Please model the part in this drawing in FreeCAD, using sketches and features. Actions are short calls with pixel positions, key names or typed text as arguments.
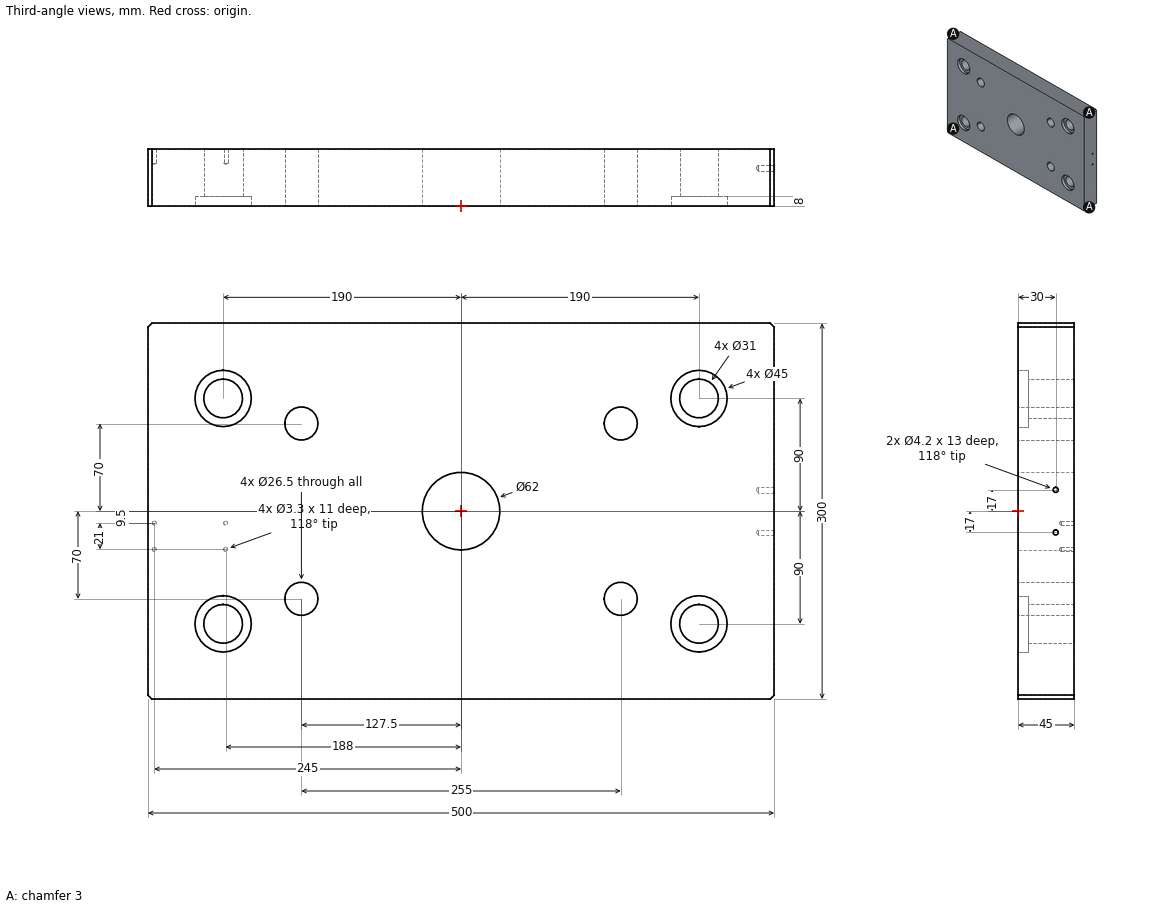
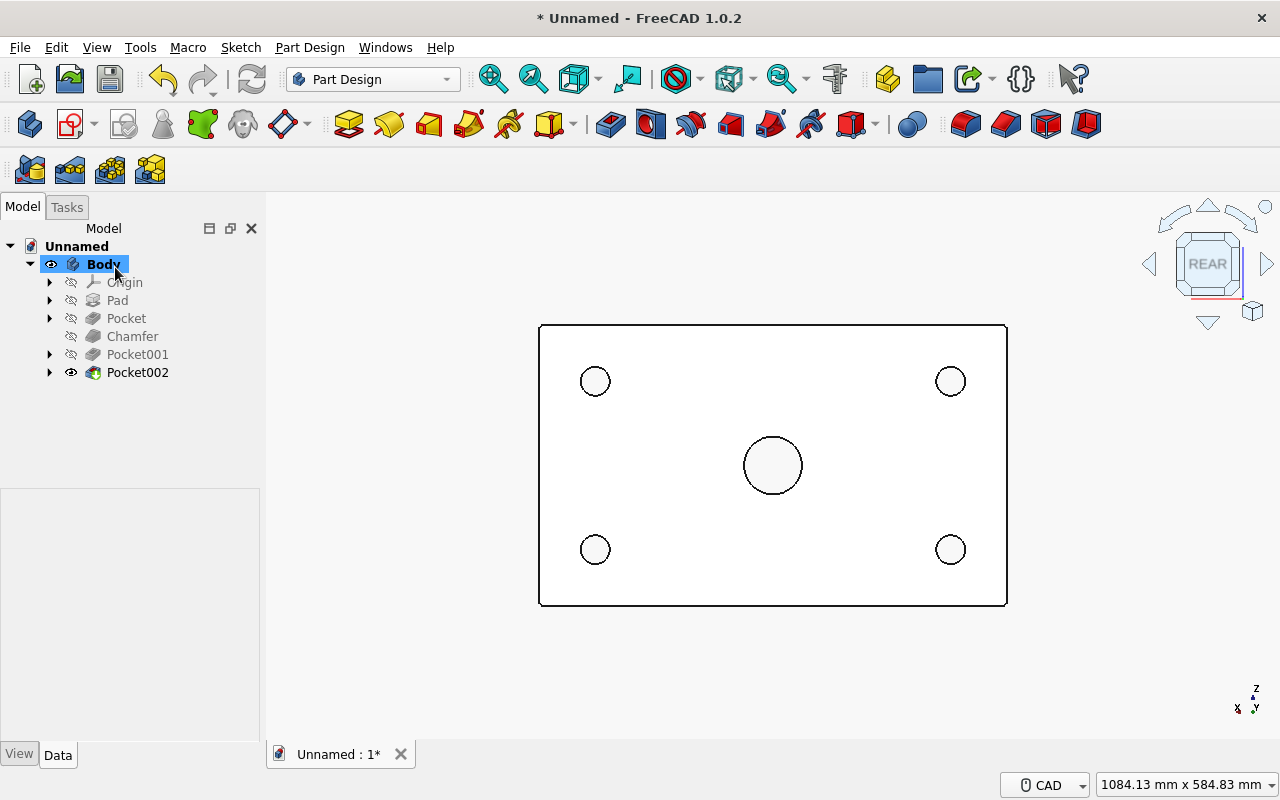
click(907, 465)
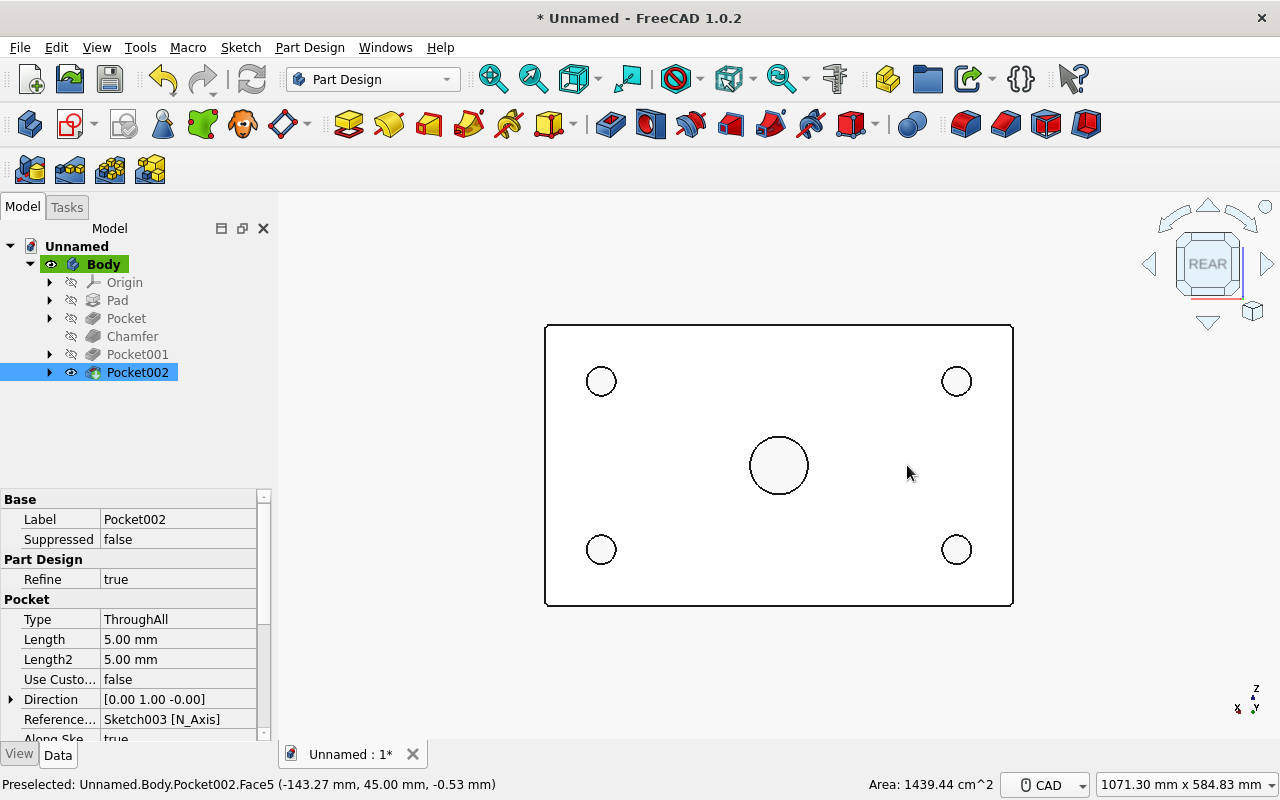
click(70, 124)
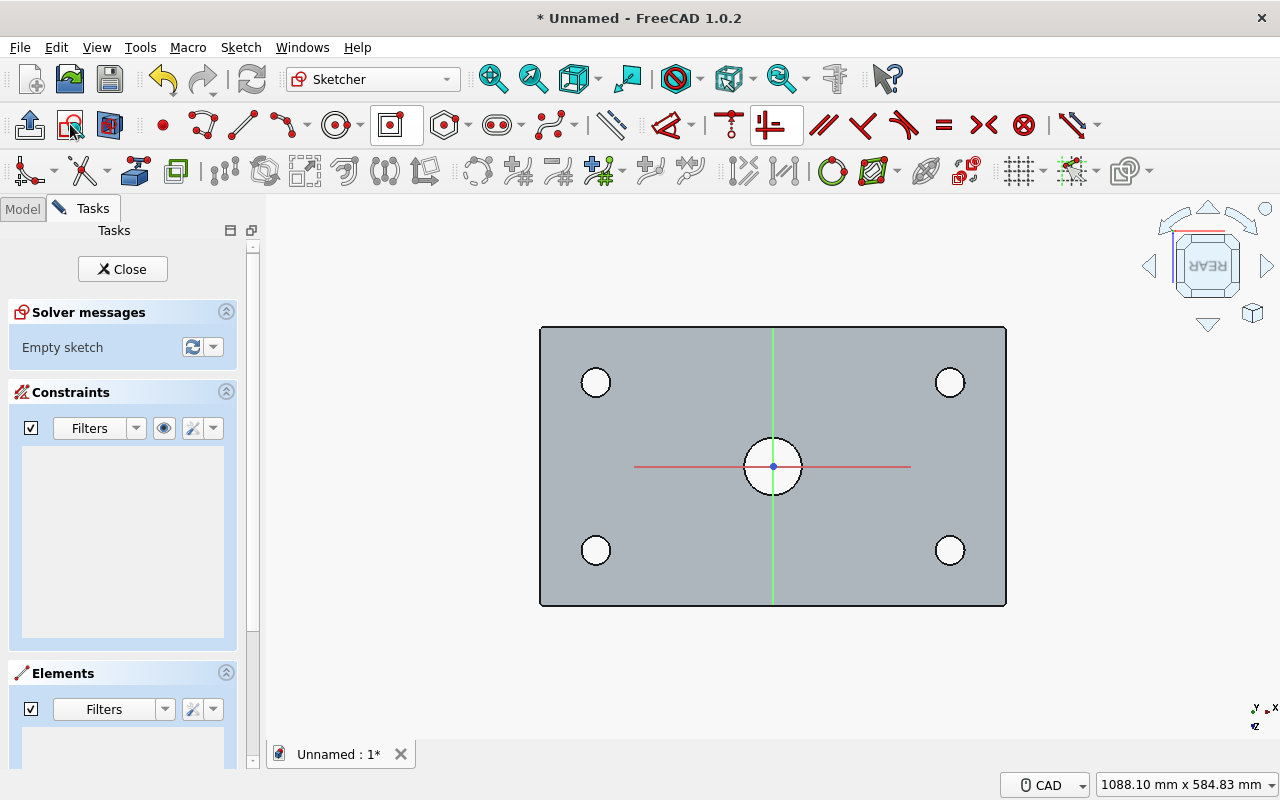
scroll(558, 446, up, 12)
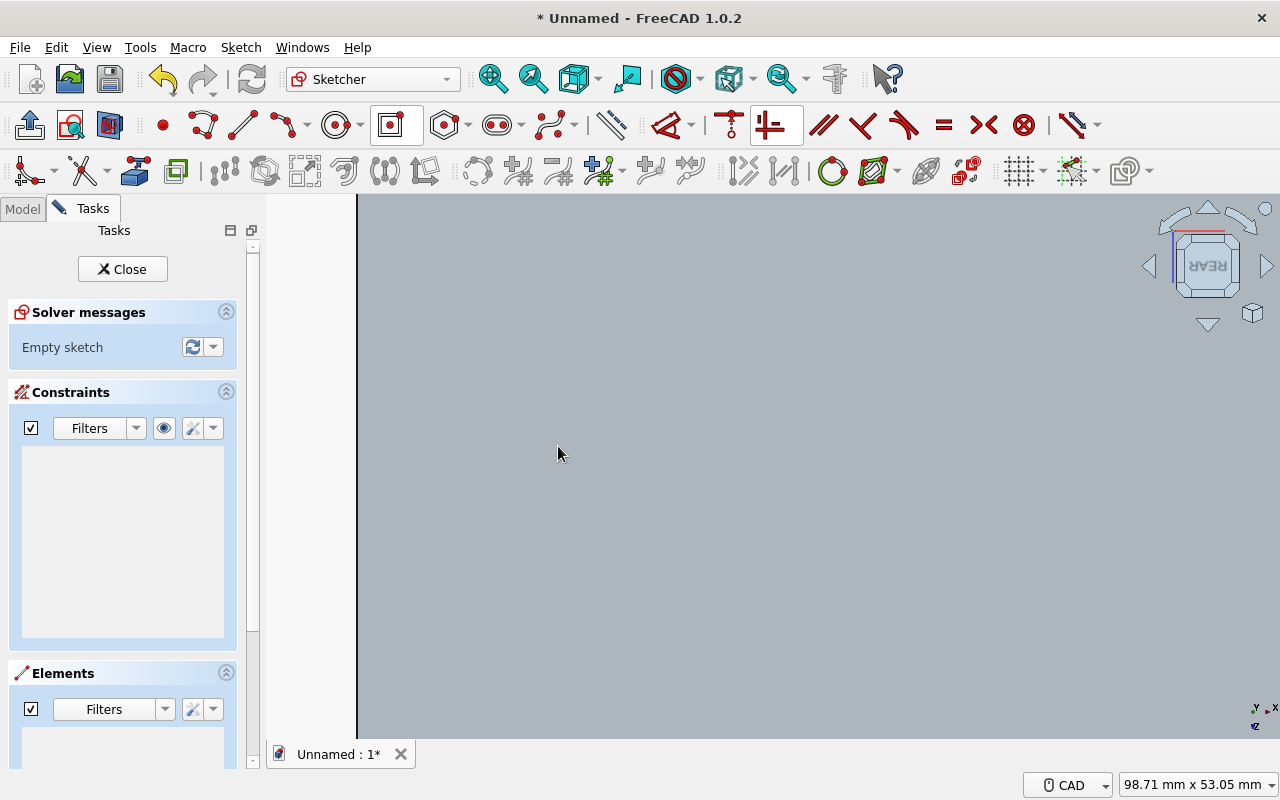
click(336, 126)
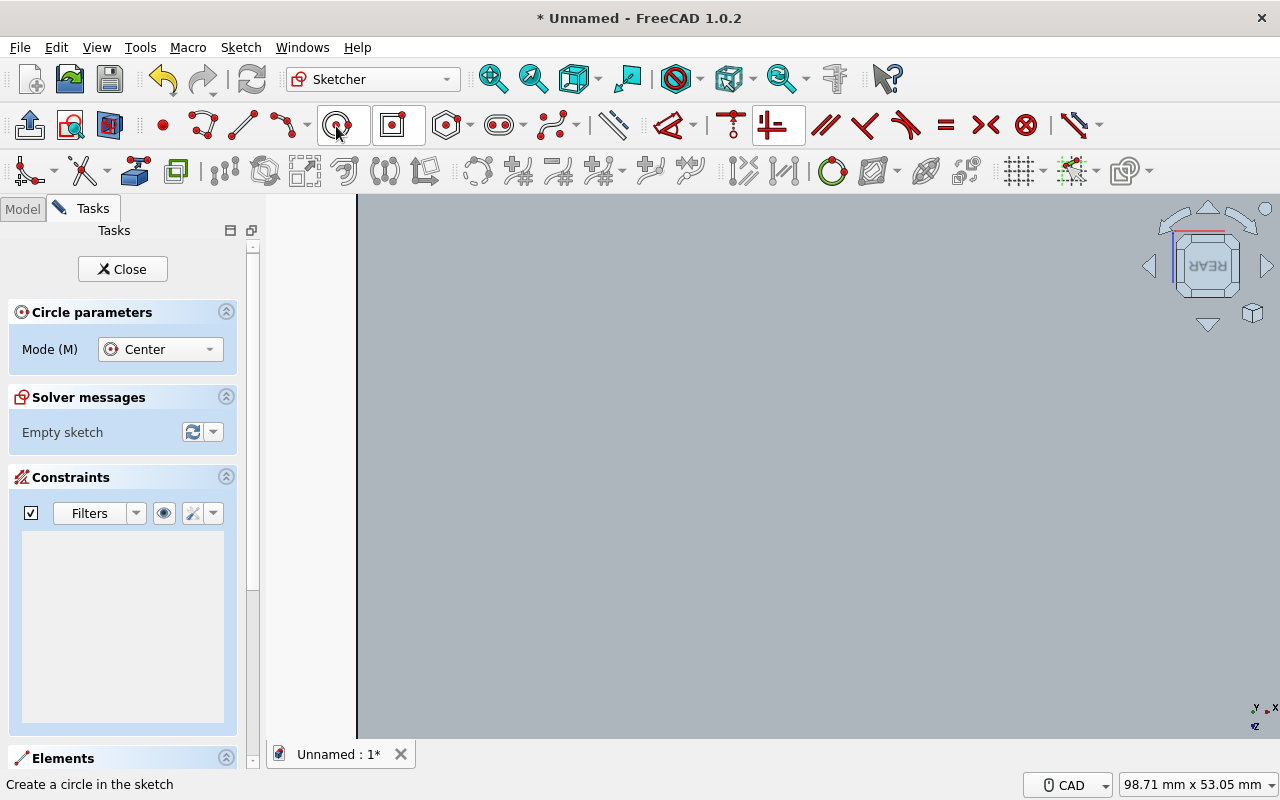
scroll(994, 354, up, 2)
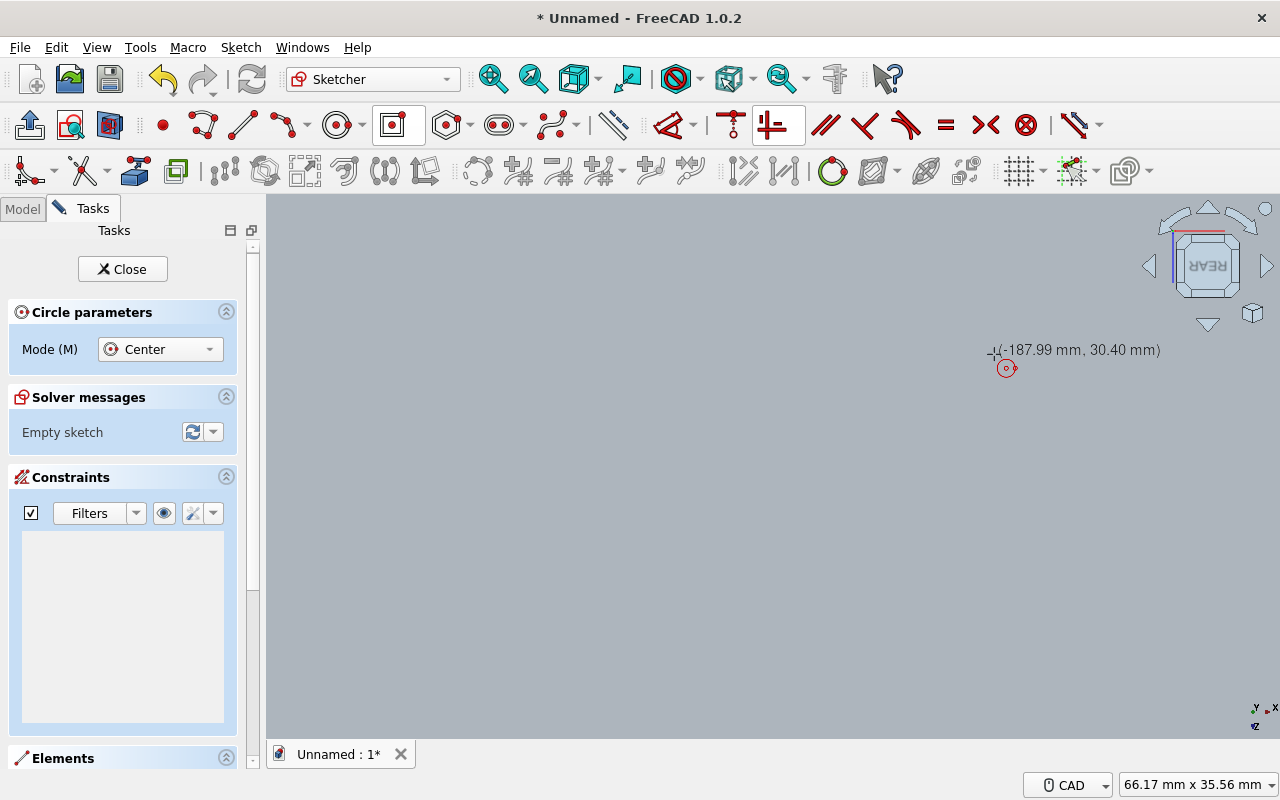
click(993, 354)
click(1011, 336)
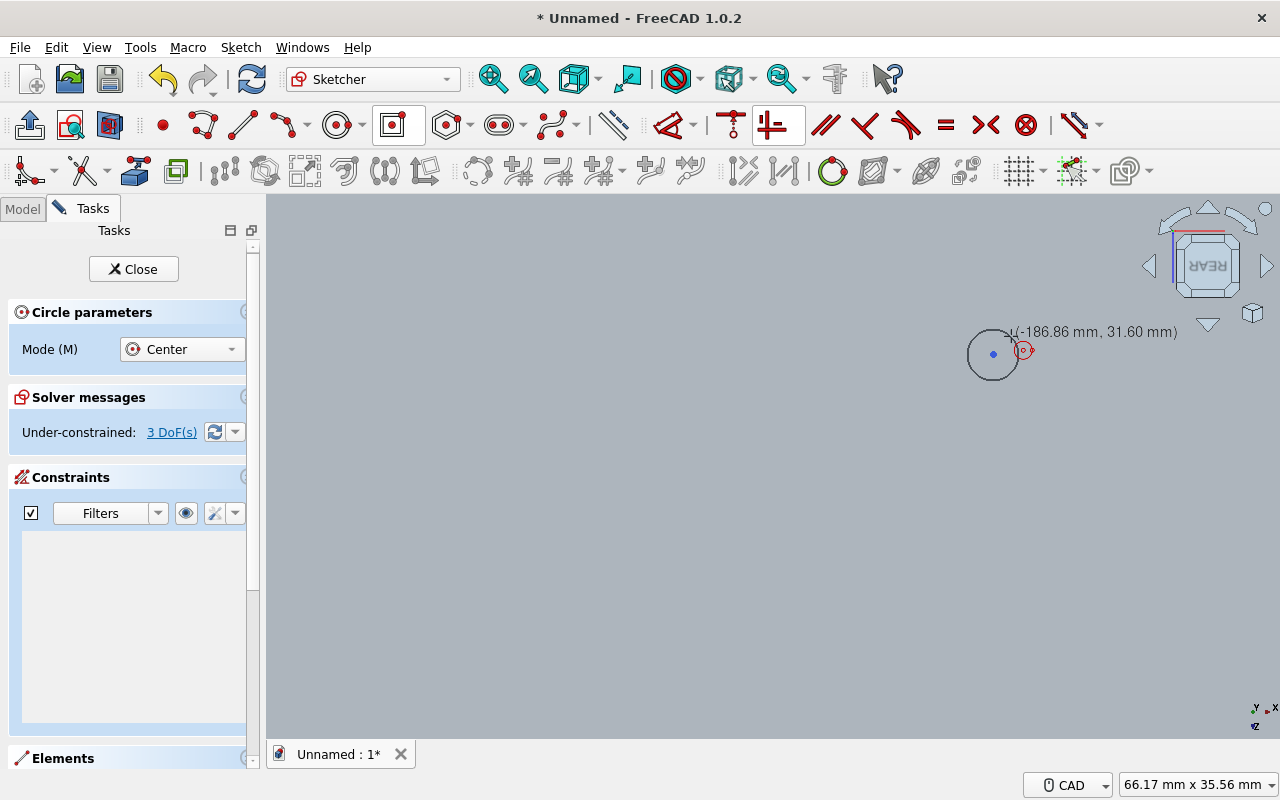
scroll(1005, 368, down, 2)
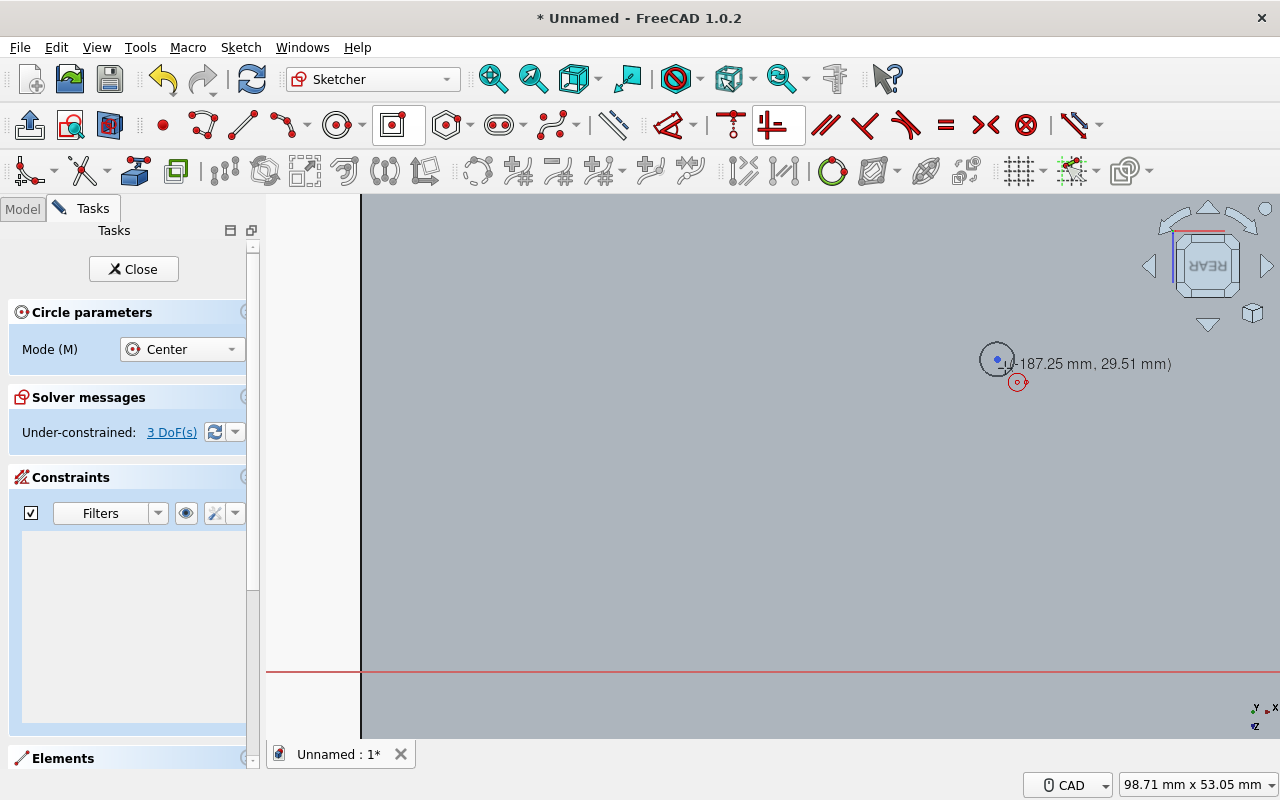
scroll(412, 574, up, 2)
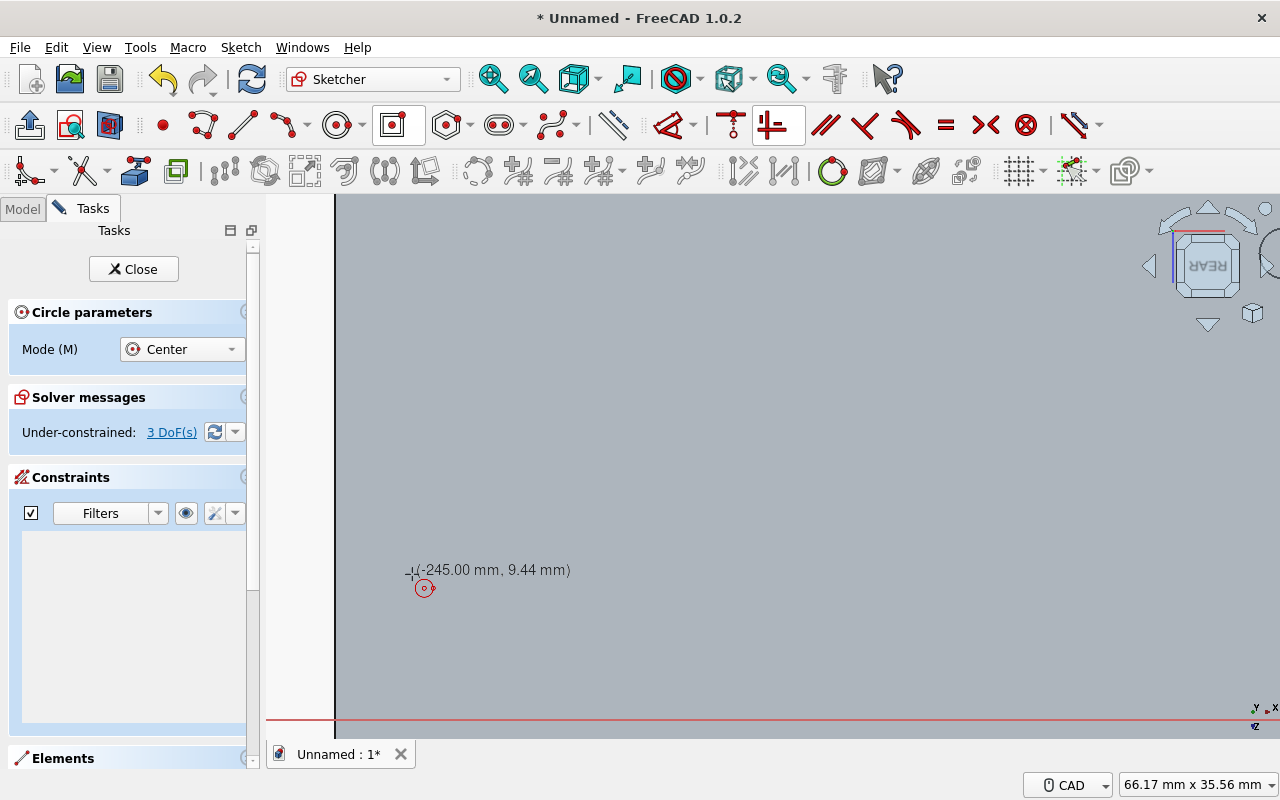
click(412, 574)
click(430, 556)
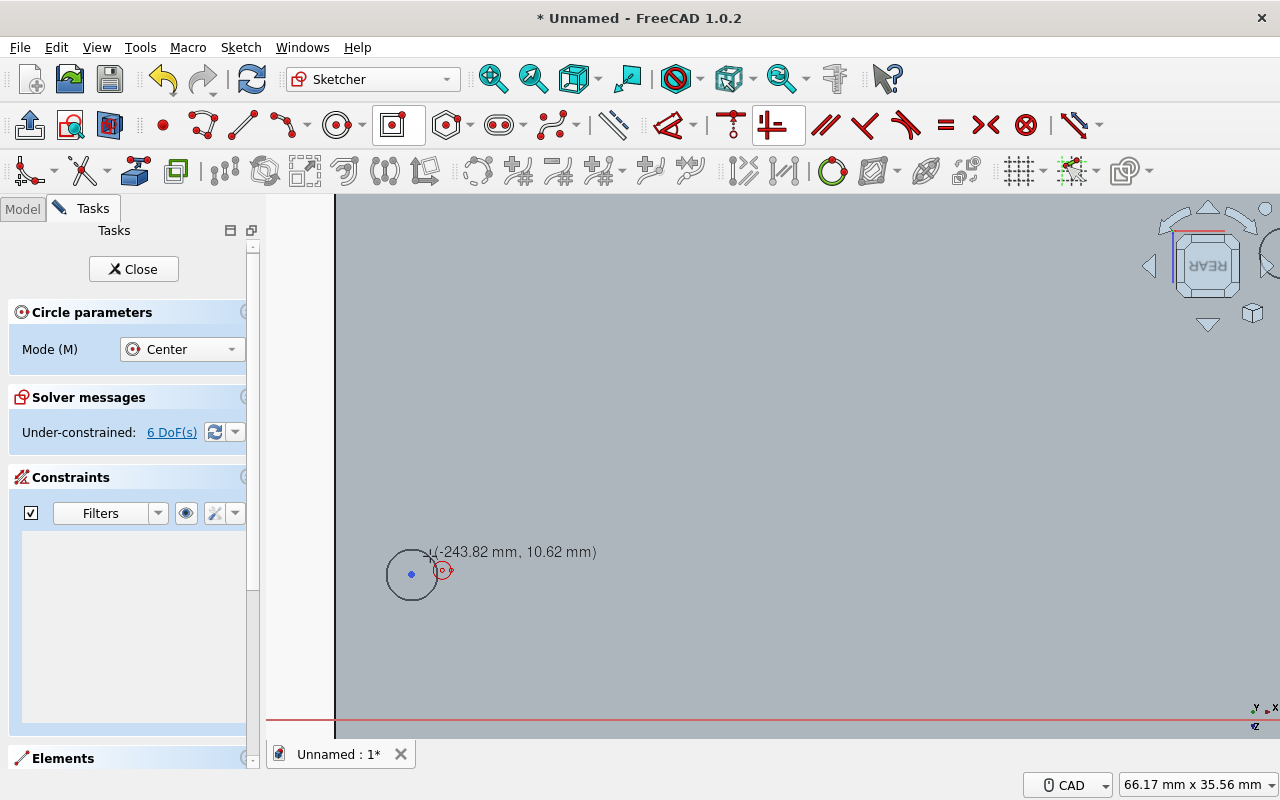
scroll(411, 575, down, 2)